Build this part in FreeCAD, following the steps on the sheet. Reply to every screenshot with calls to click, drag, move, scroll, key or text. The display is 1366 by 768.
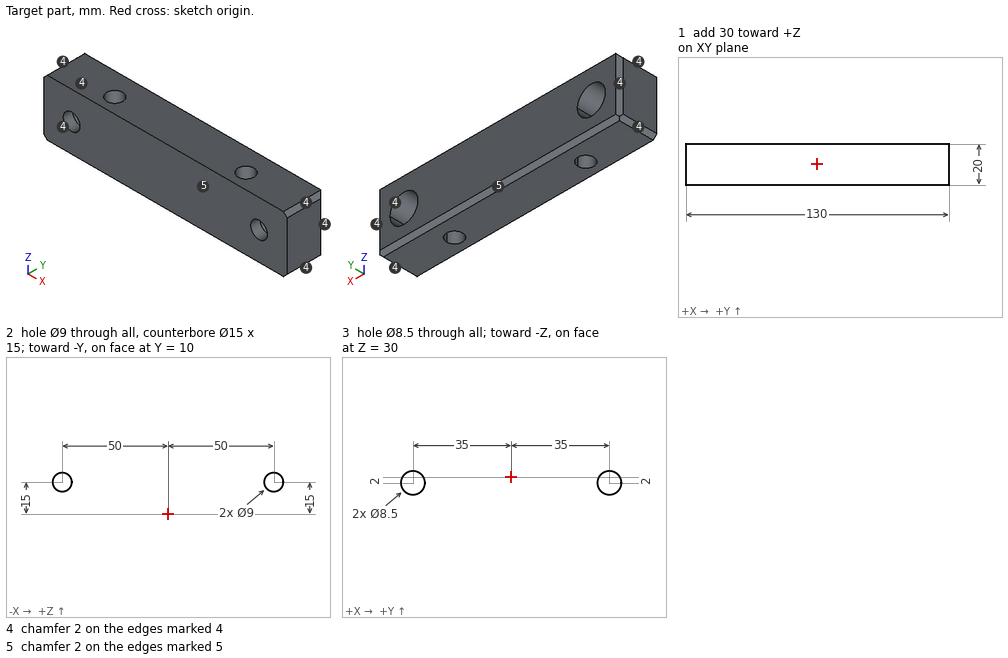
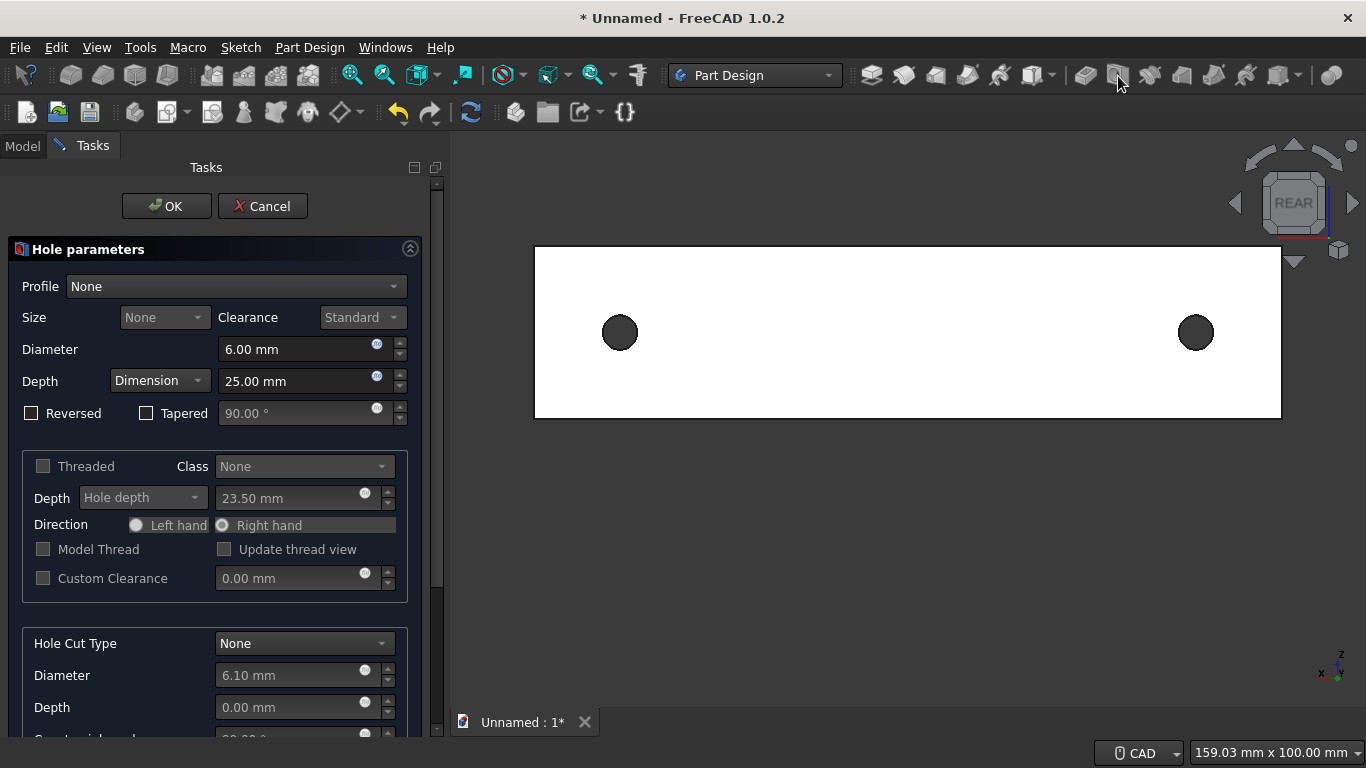
triple_click(305, 349)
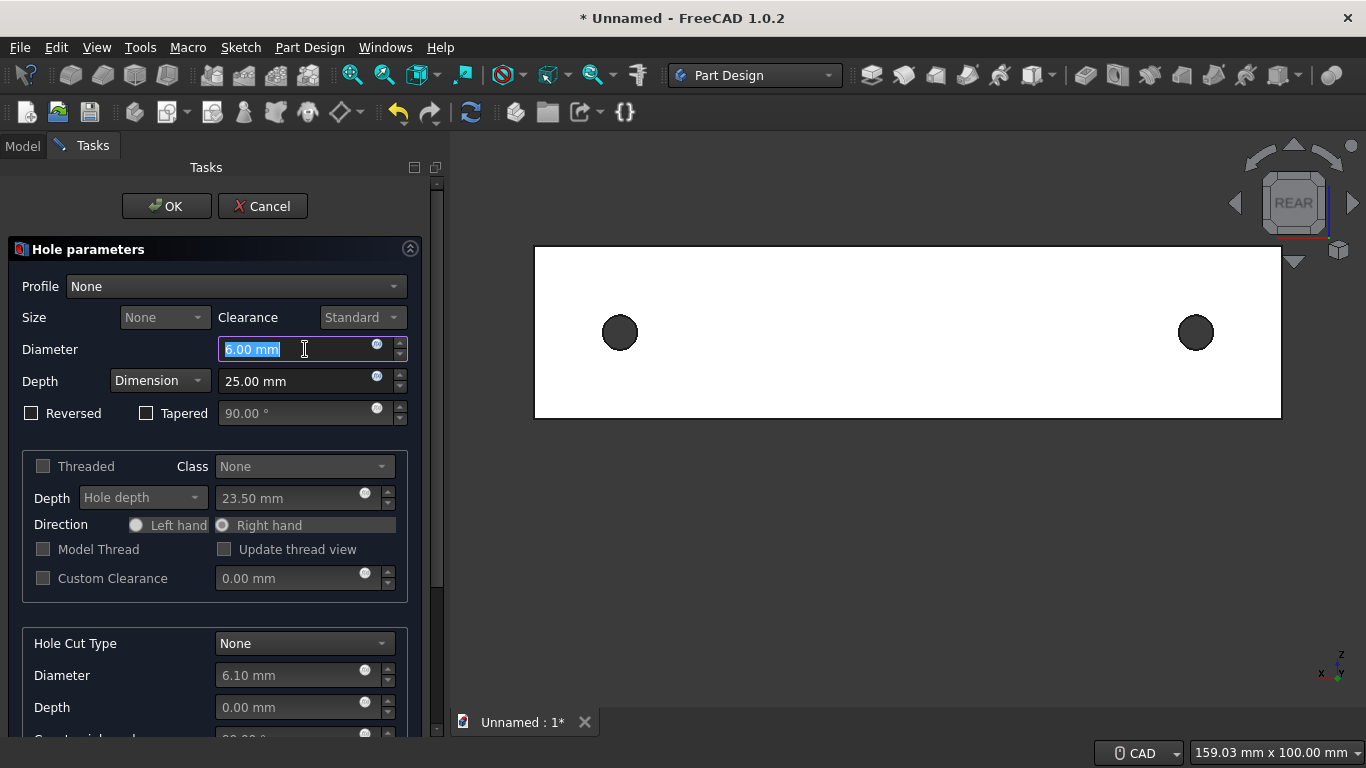
text(9)
key(Tab)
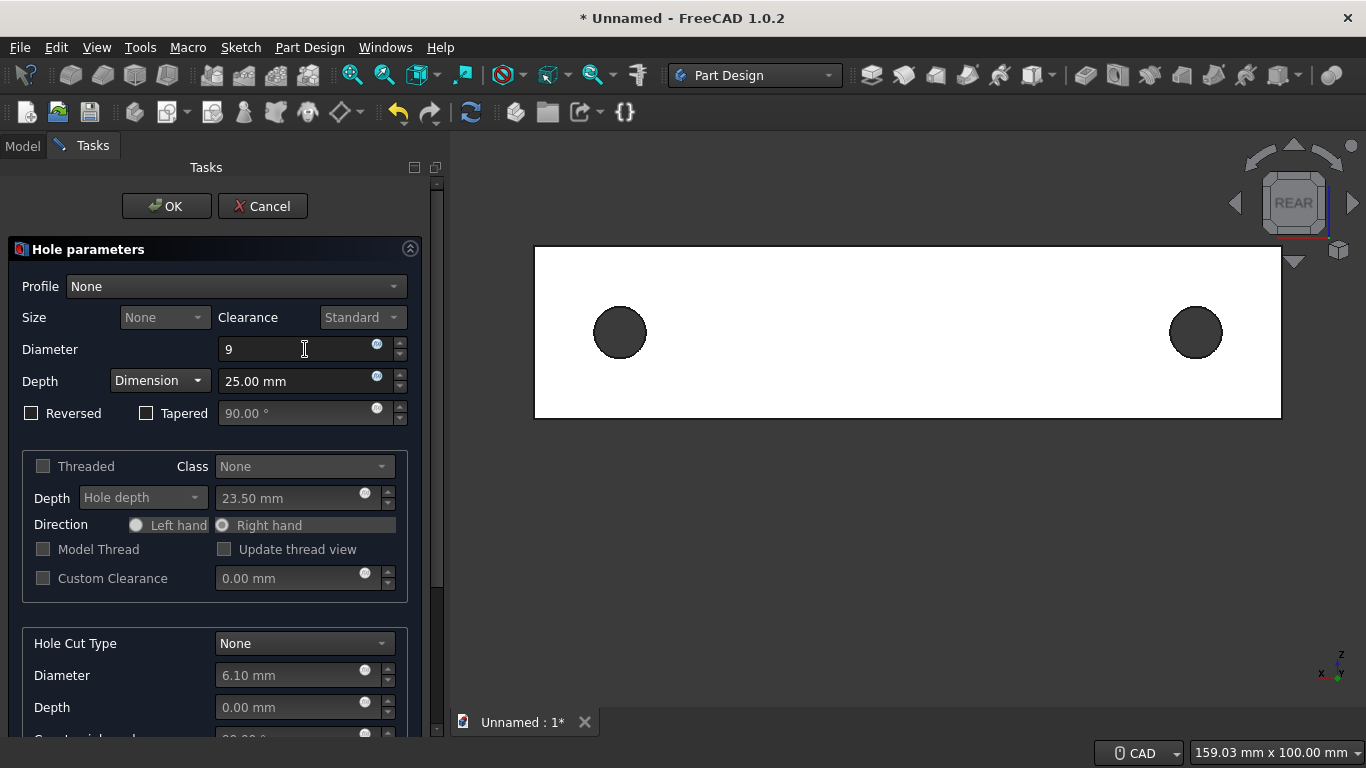
click(161, 380)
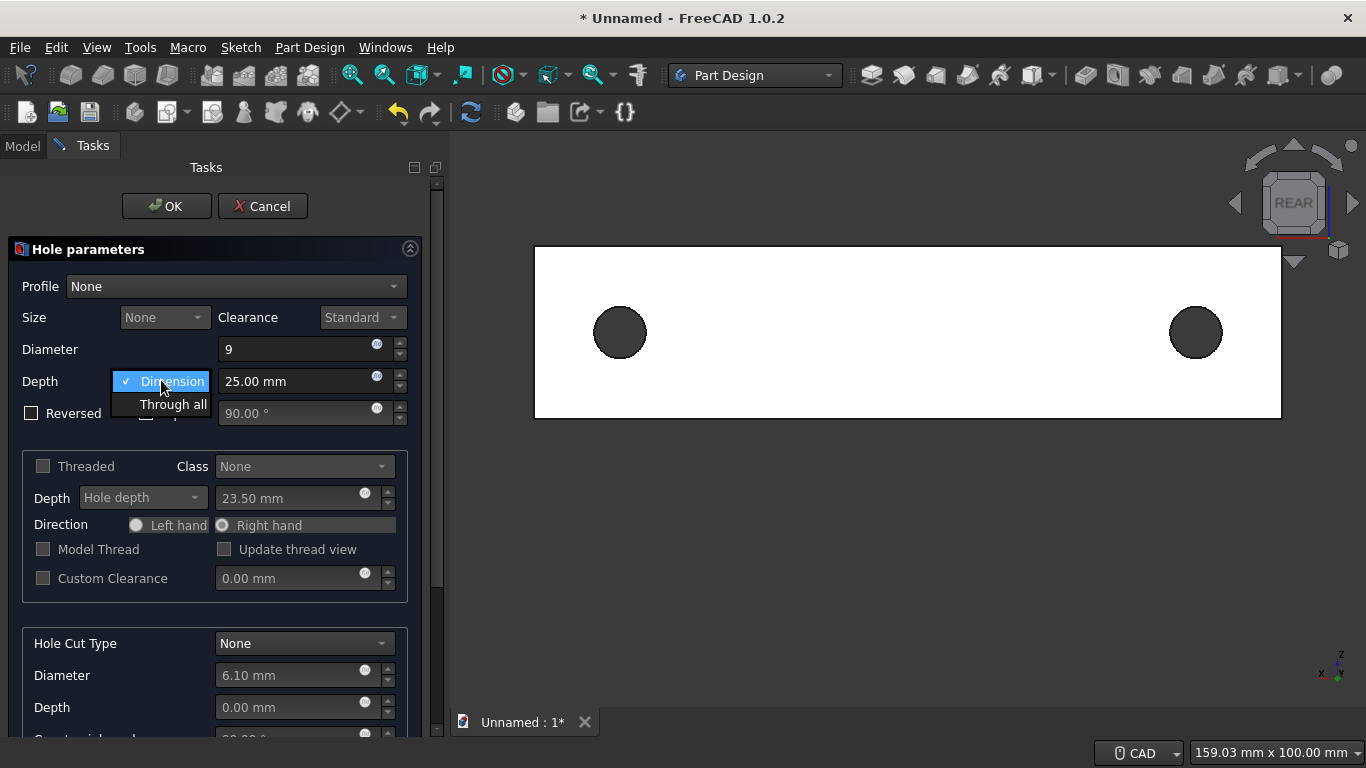
click(160, 404)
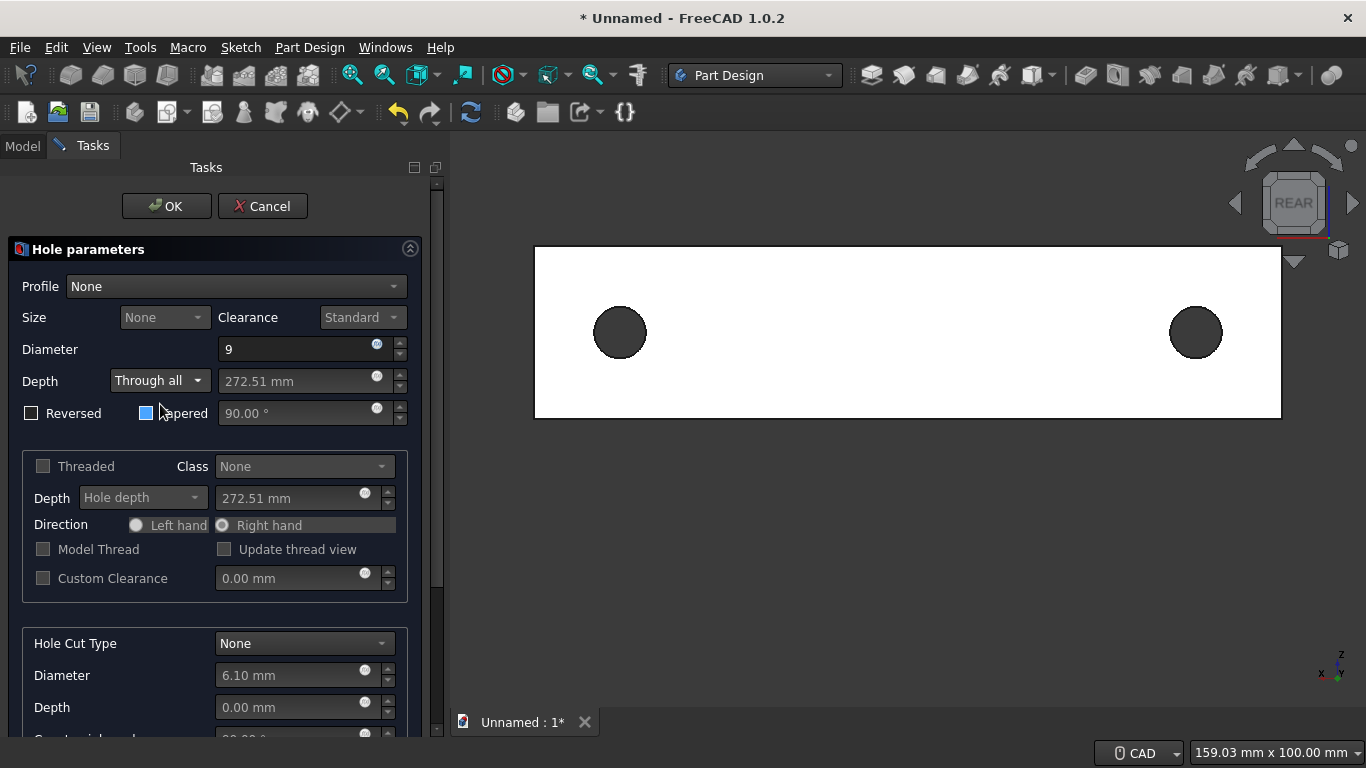
click(306, 644)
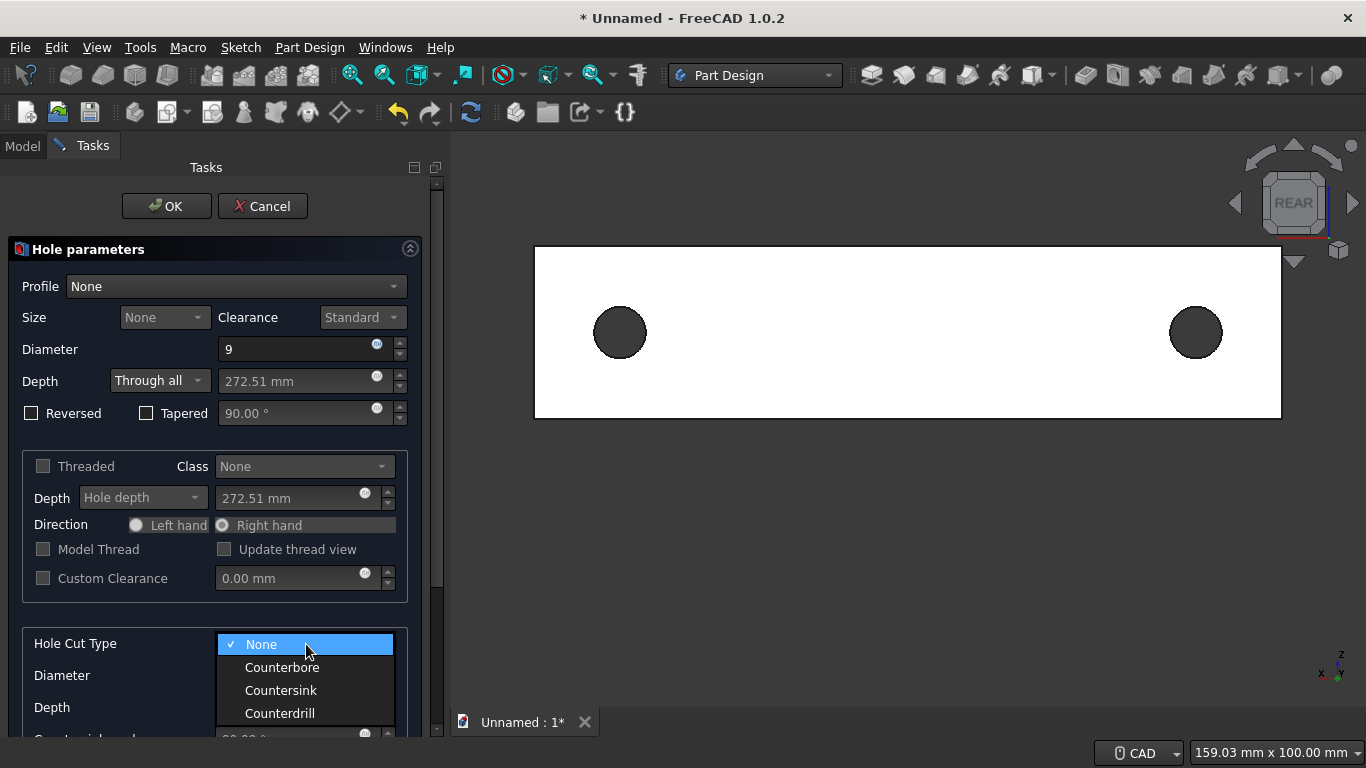
click(304, 668)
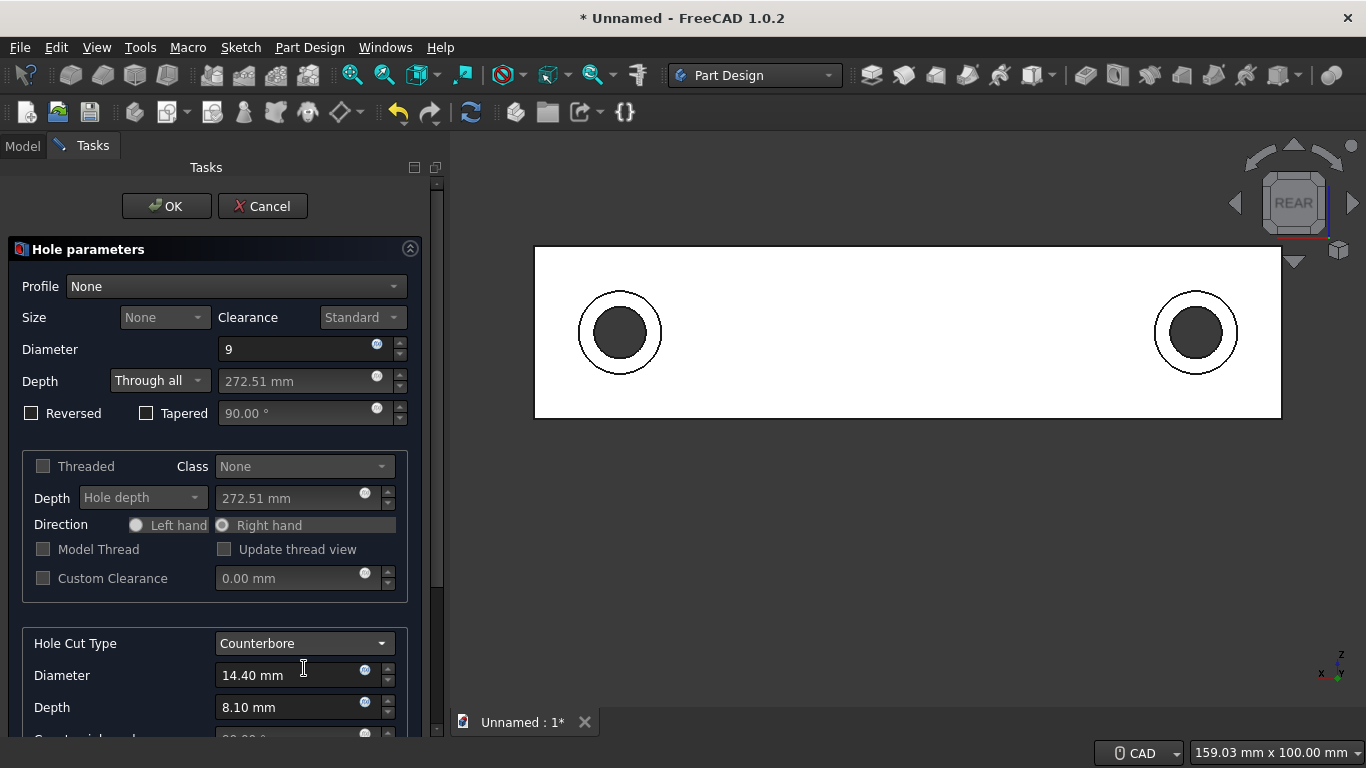
triple_click(298, 675)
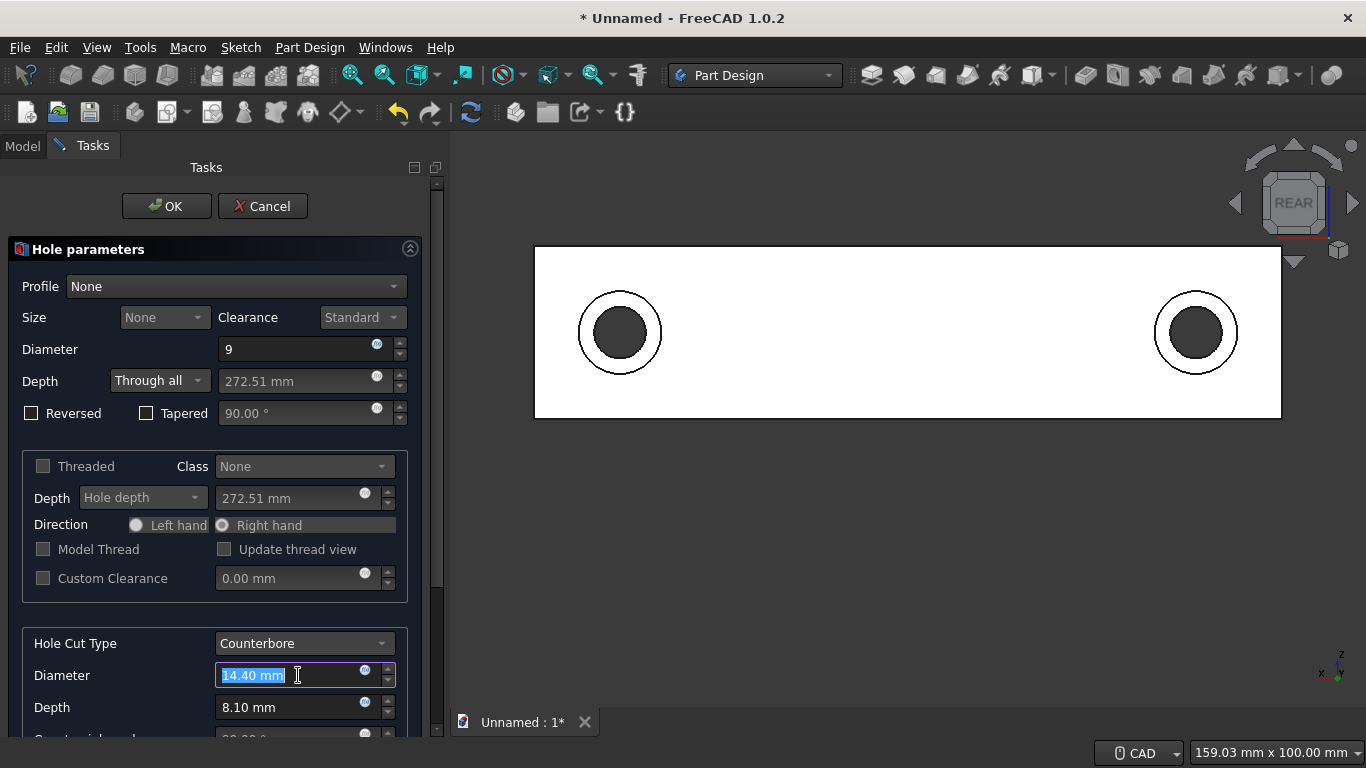
text(15)
key(Tab)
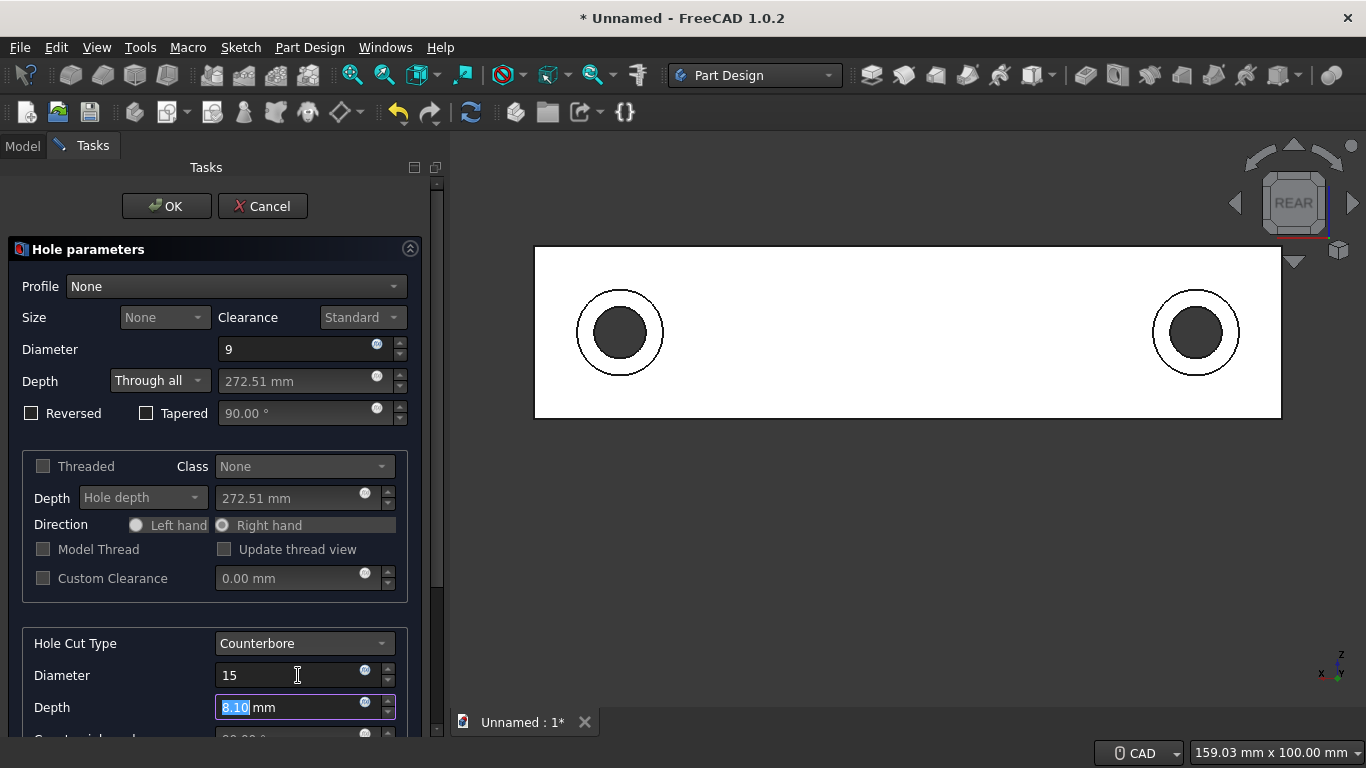
text(15)
key(Tab)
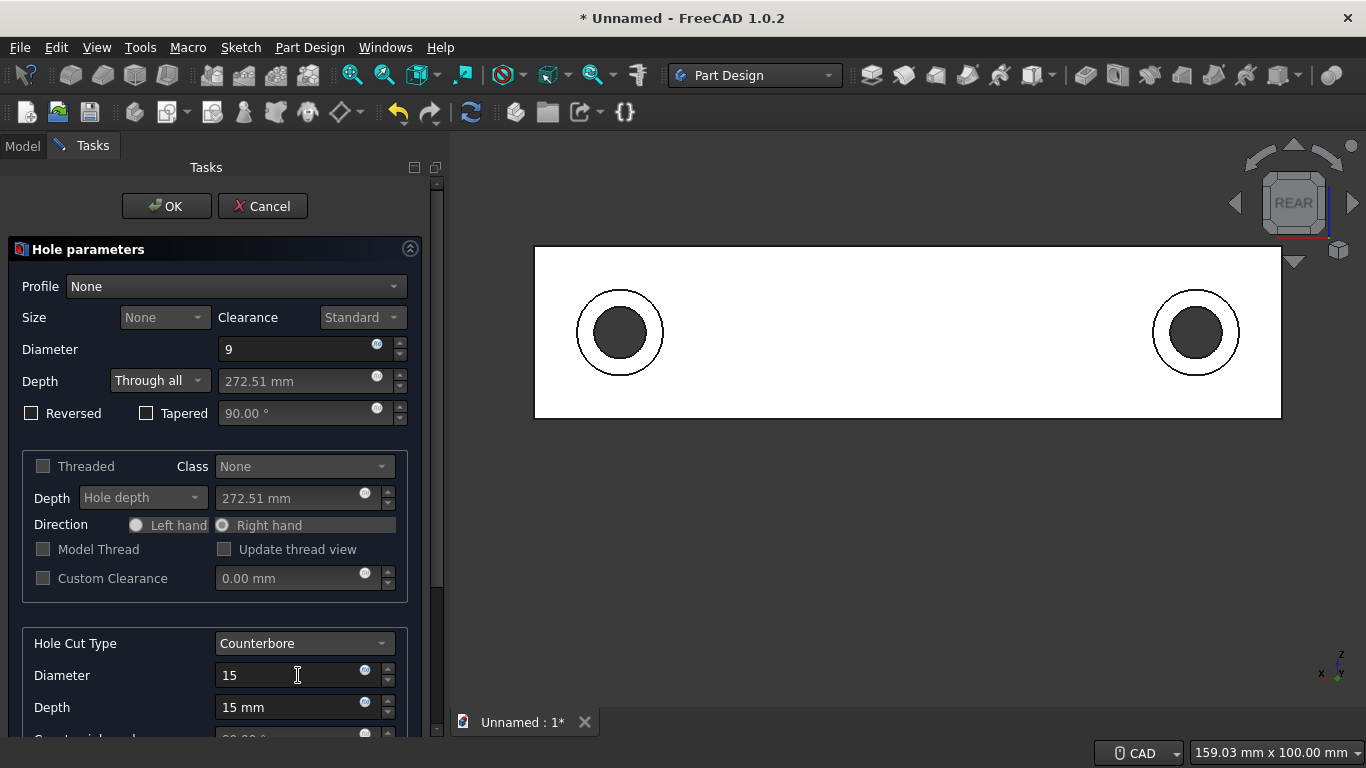
click(167, 206)